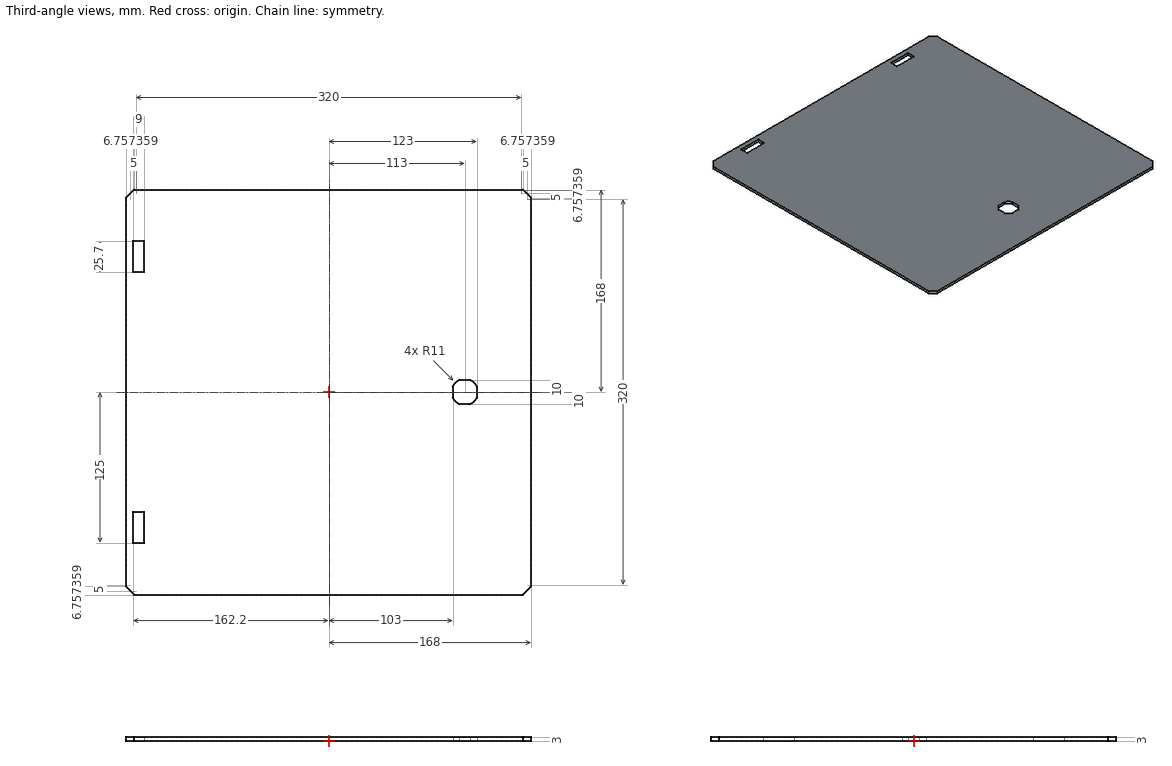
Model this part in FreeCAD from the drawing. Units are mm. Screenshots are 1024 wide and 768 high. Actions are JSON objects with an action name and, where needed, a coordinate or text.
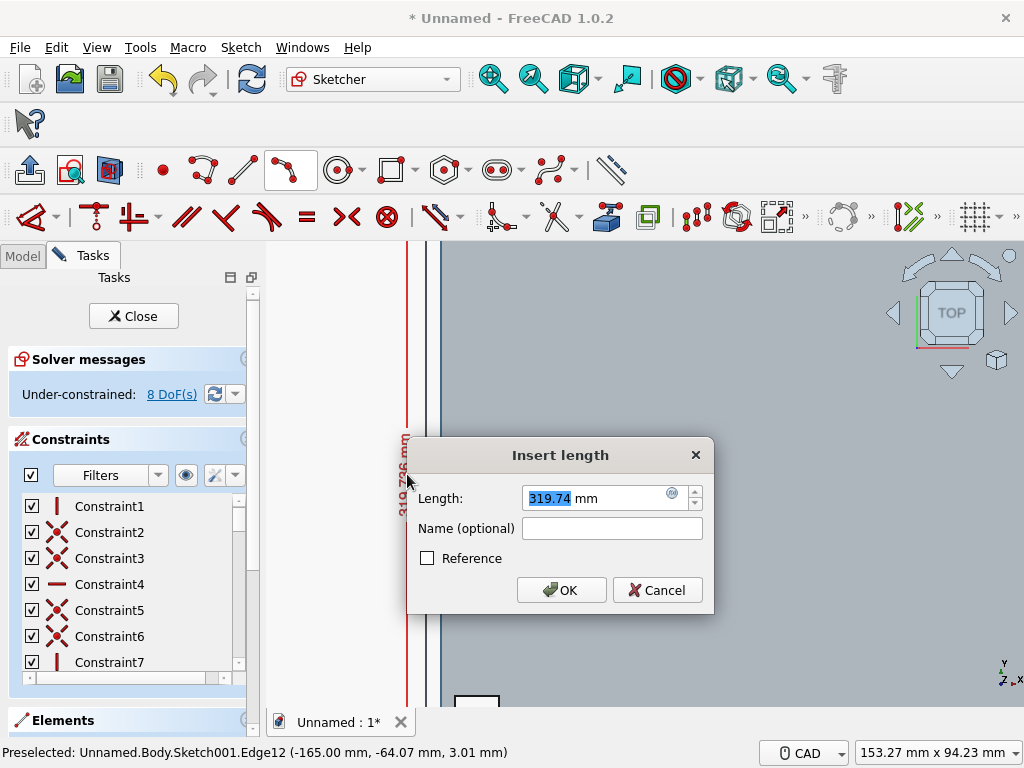
{"action": "type", "text": "320"}
{"action": "key", "text": "Return"}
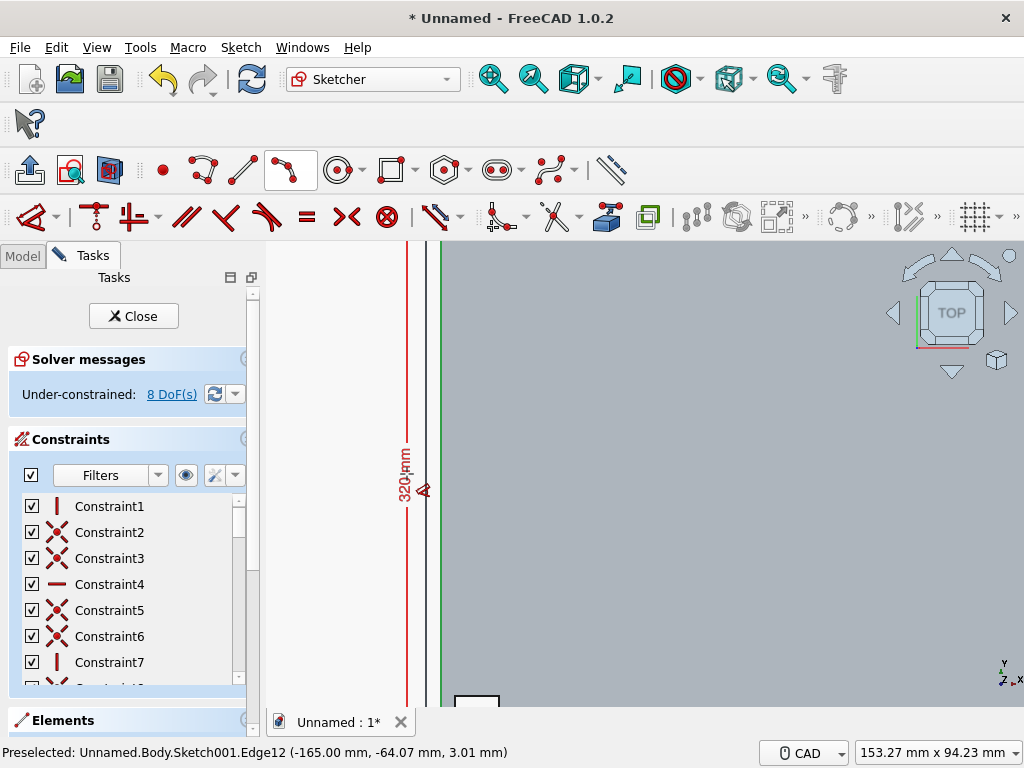
{"action": "scroll", "coordinate": [442, 527], "scroll_direction": "down", "scroll_amount": 9}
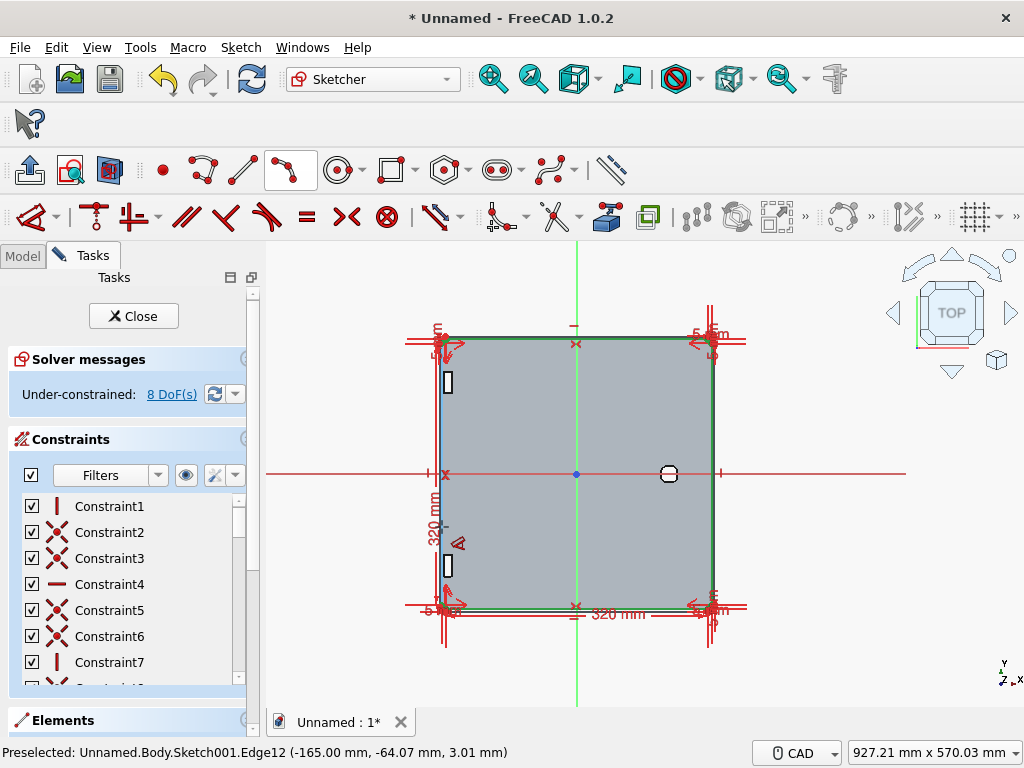
{"action": "scroll", "coordinate": [714, 607], "scroll_direction": "up", "scroll_amount": 7}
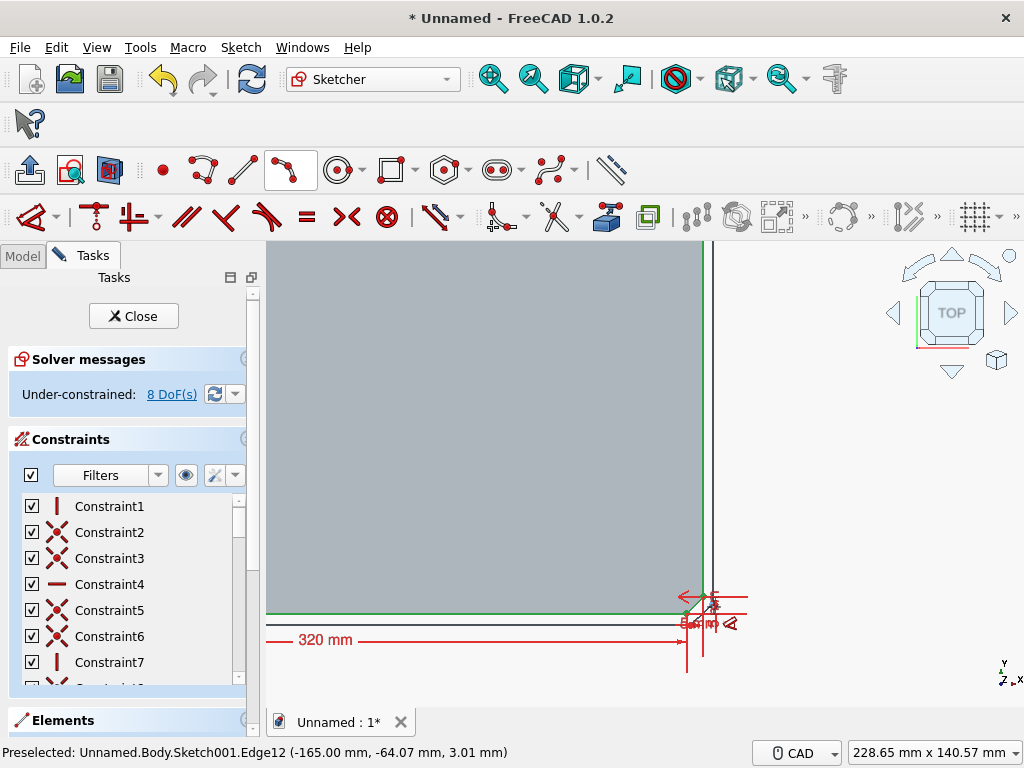
{"action": "left_click", "coordinate": [713, 604]}
{"action": "left_click", "coordinate": [503, 638]}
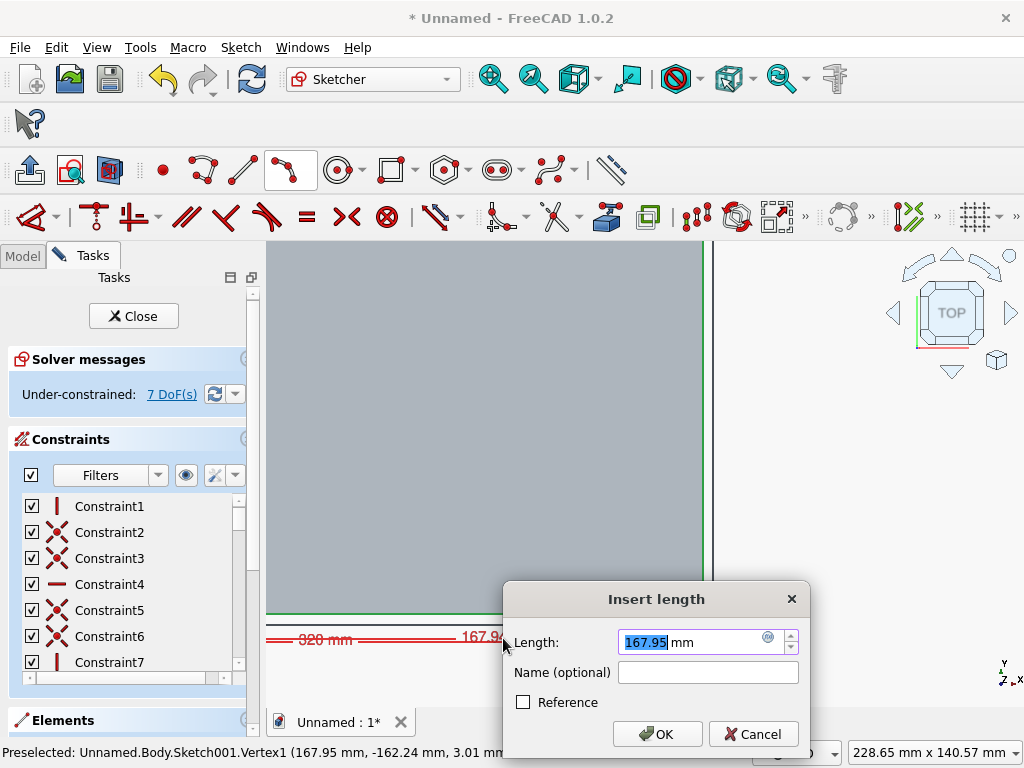
{"action": "type", "text": "168"}
{"action": "key", "text": "Return"}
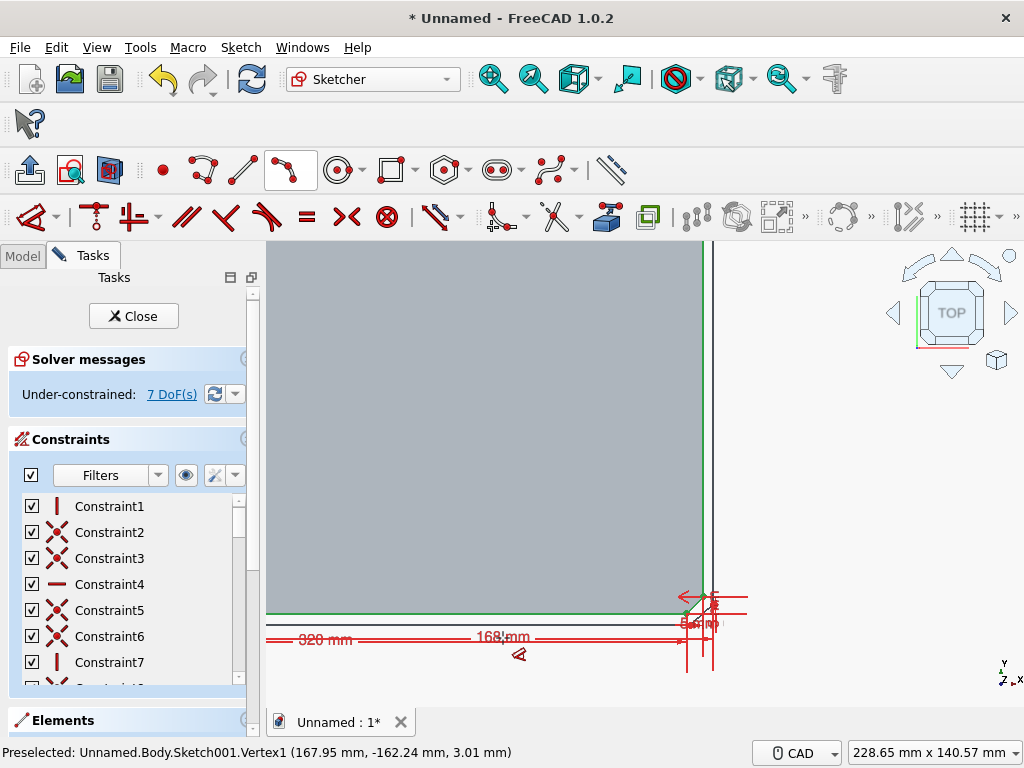
{"action": "scroll", "coordinate": [714, 607], "scroll_direction": "down", "scroll_amount": 7}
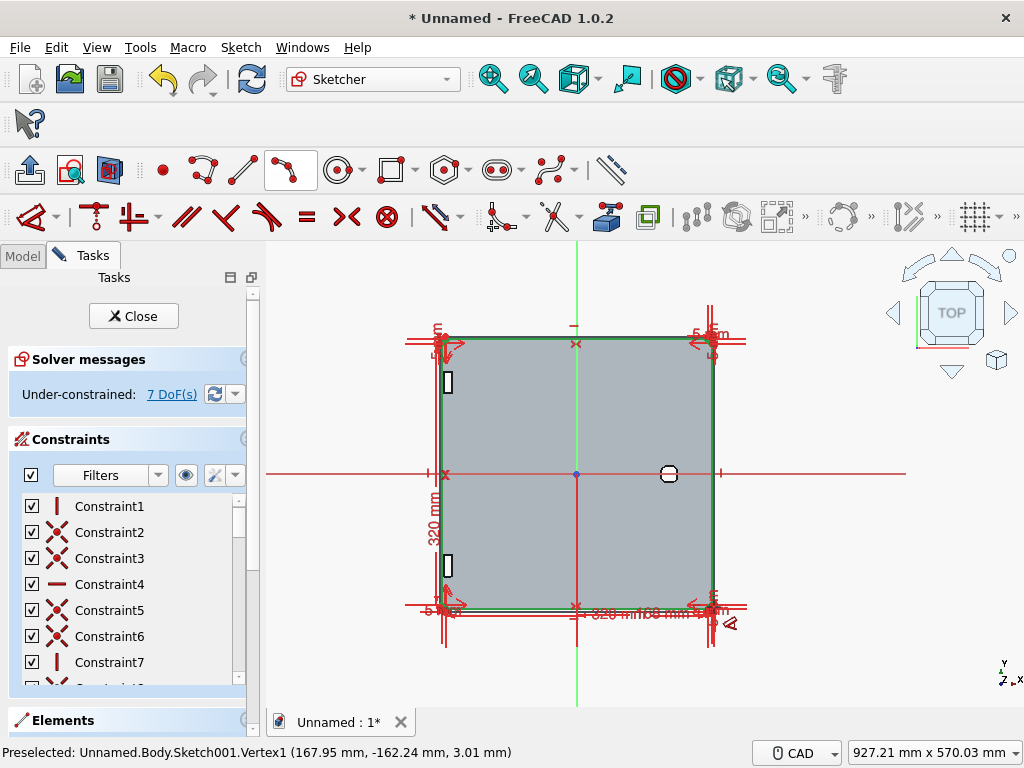
{"action": "scroll", "coordinate": [709, 337], "scroll_direction": "up", "scroll_amount": 8}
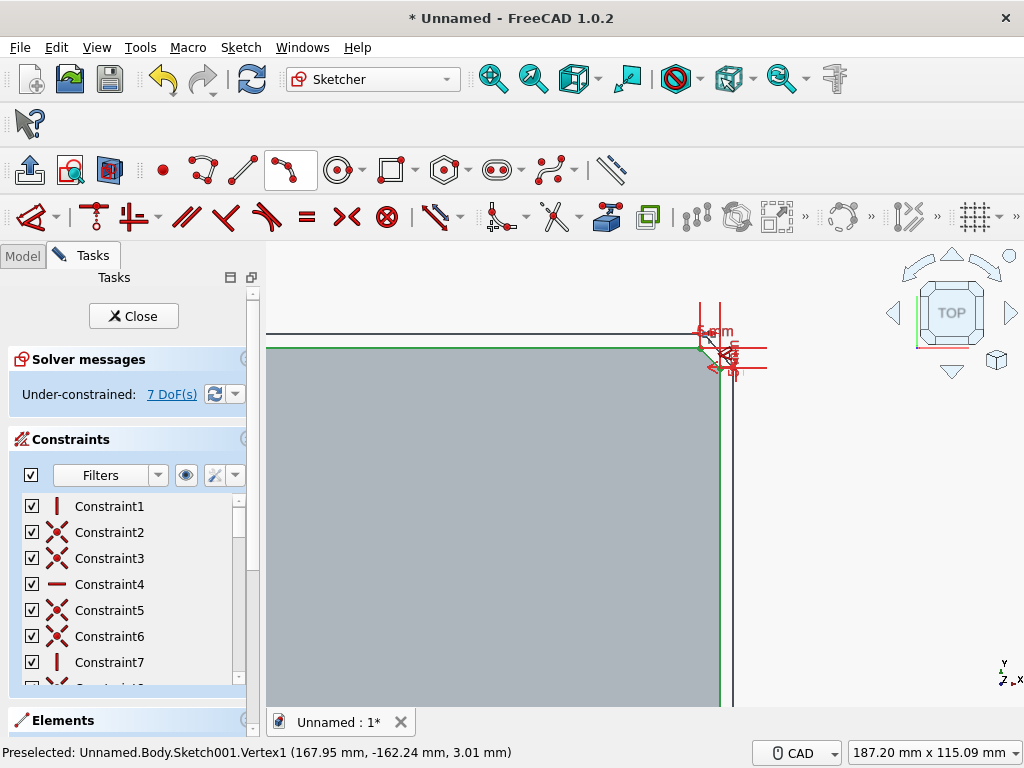
{"action": "left_click", "coordinate": [704, 334]}
{"action": "left_click", "coordinate": [762, 507]}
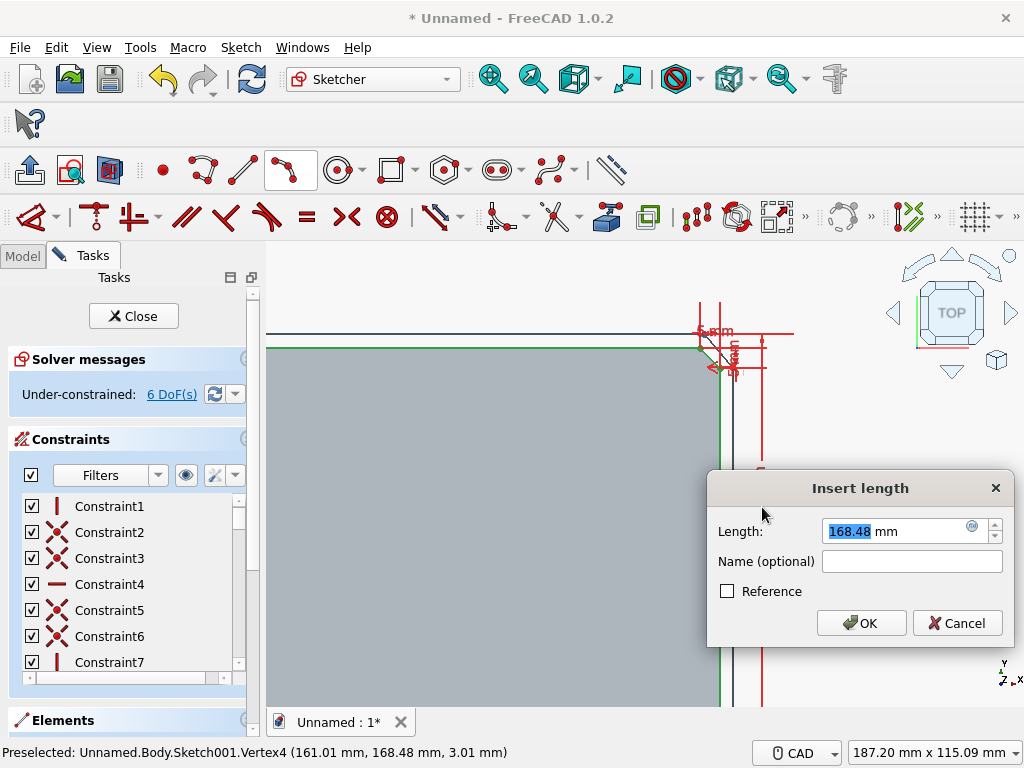
{"action": "type", "text": "168"}
{"action": "key", "text": "Return"}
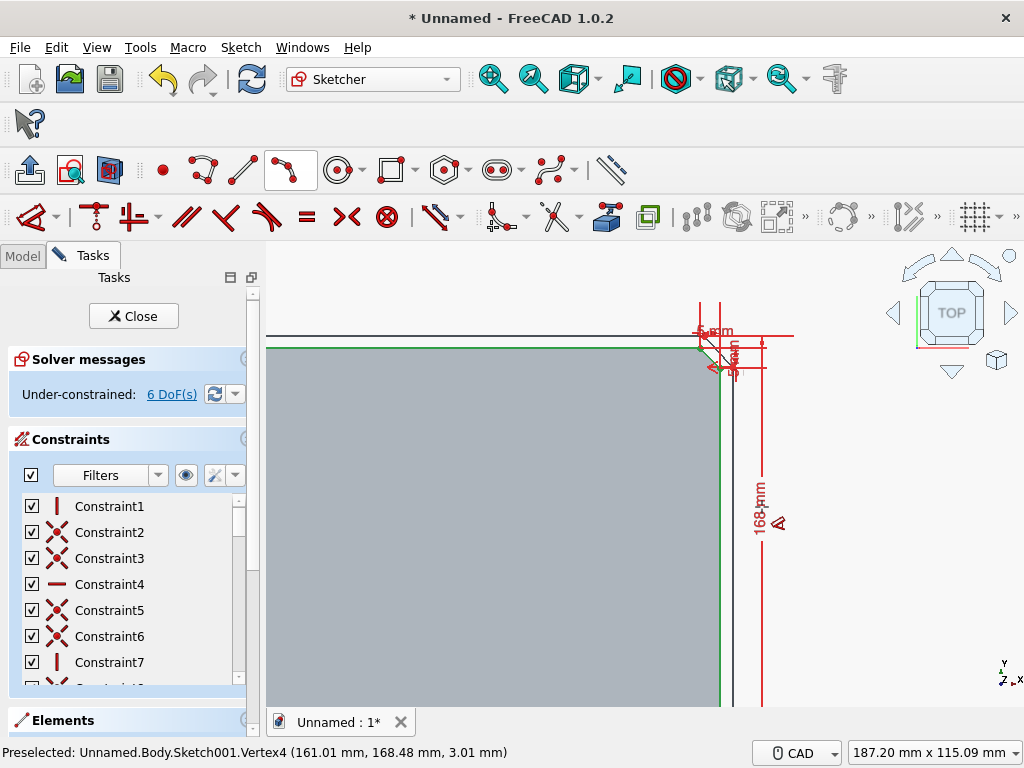
{"action": "scroll", "coordinate": [724, 358], "scroll_direction": "up", "scroll_amount": 2}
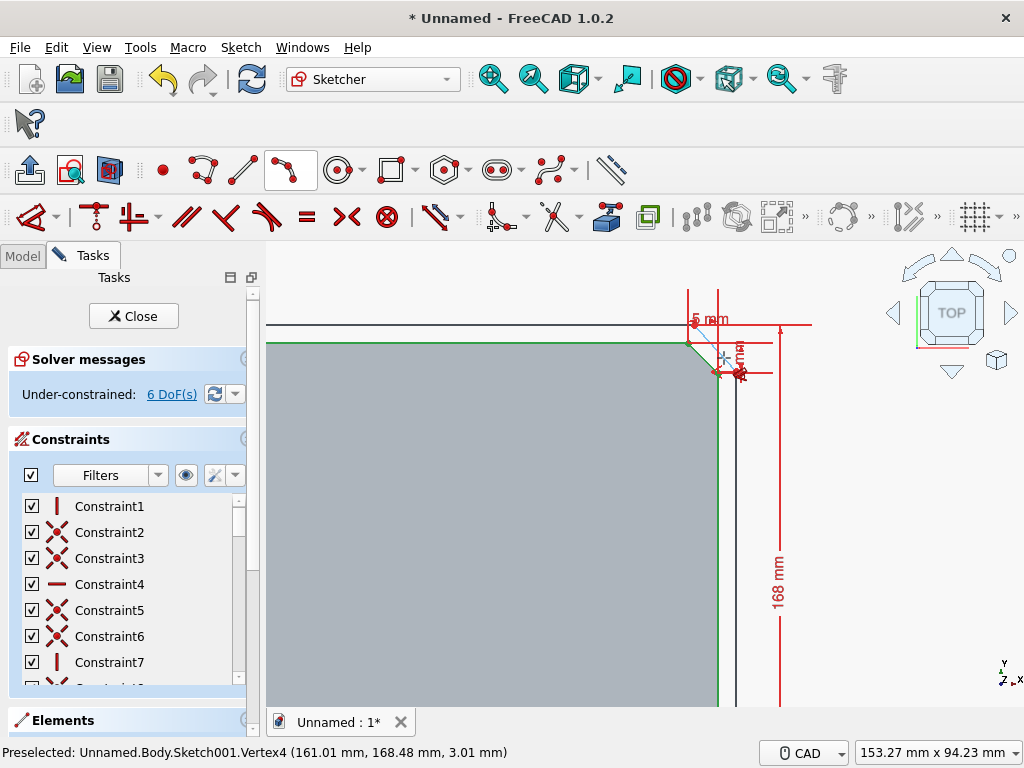
{"action": "left_click", "coordinate": [724, 358]}
{"action": "left_click", "coordinate": [715, 291]}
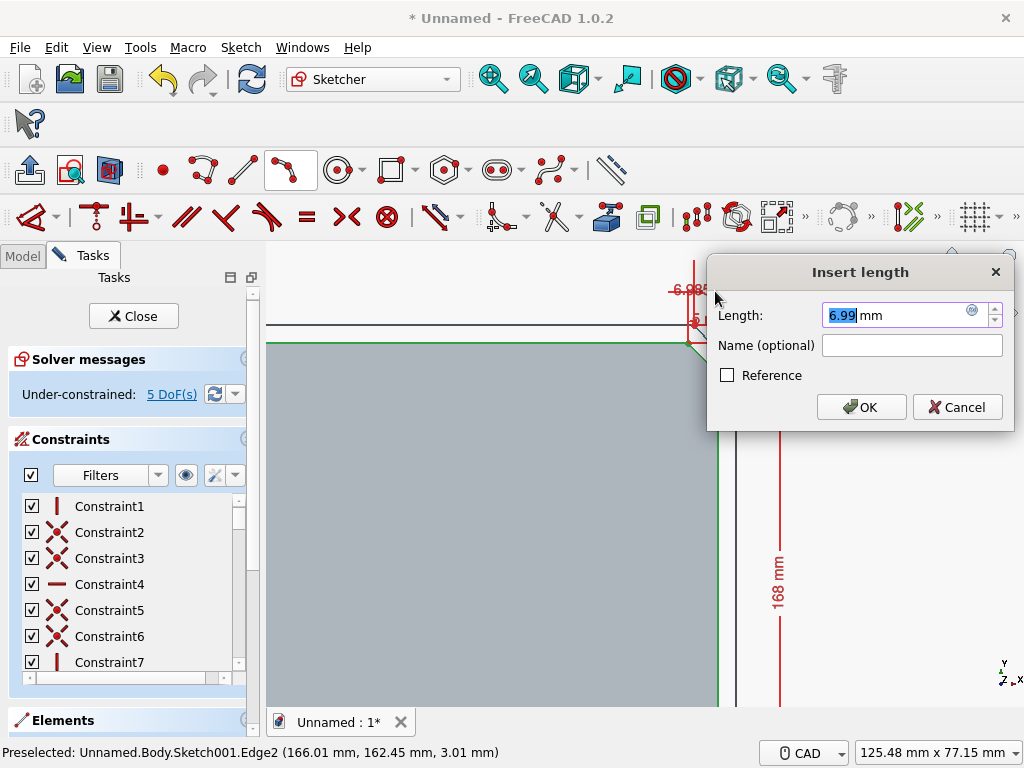
{"action": "type", "text": "6.757359"}
{"action": "key", "text": "Return"}